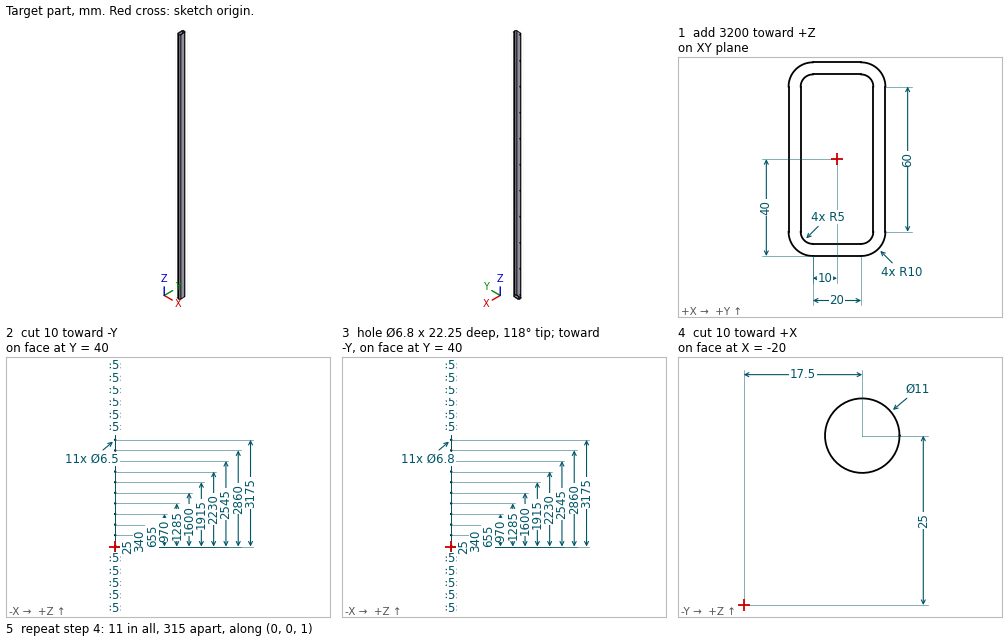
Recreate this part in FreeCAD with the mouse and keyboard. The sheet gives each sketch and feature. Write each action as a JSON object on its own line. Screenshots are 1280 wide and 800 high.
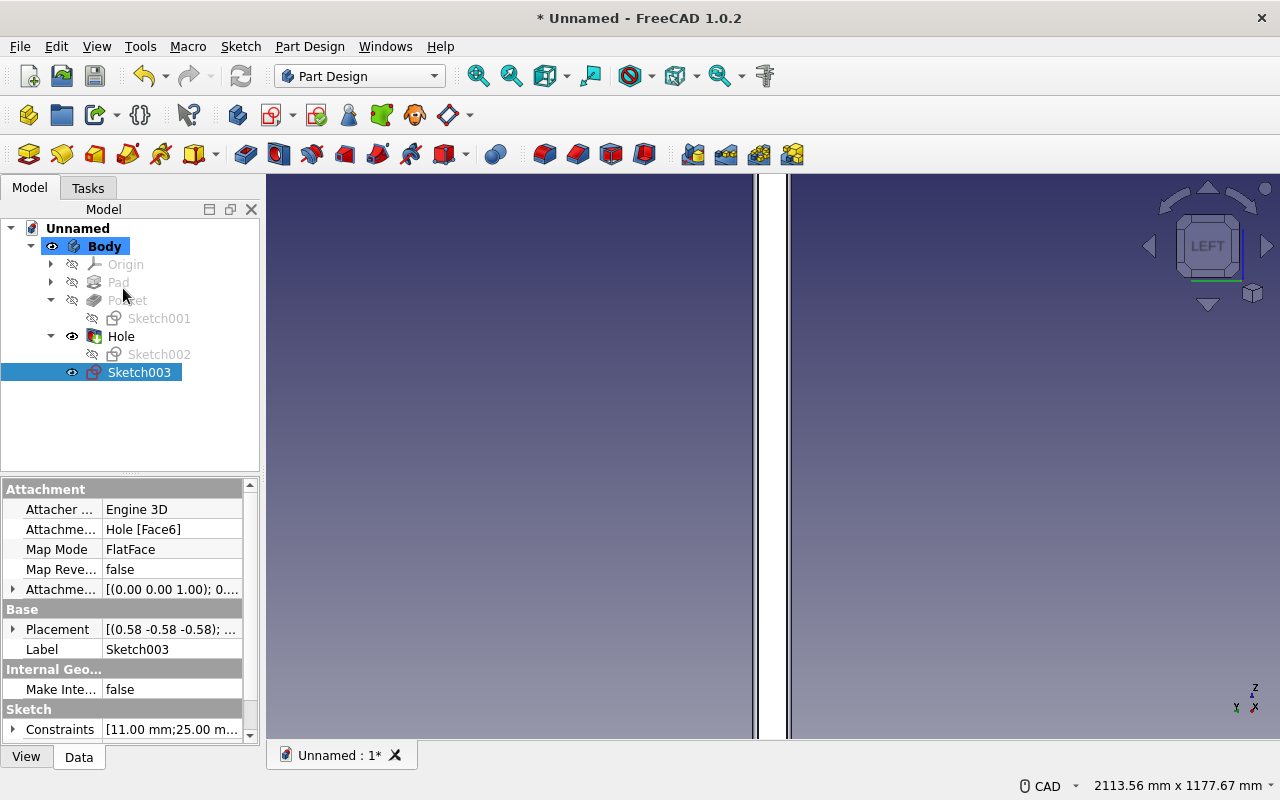
{"action": "left_click", "coordinate": [246, 154]}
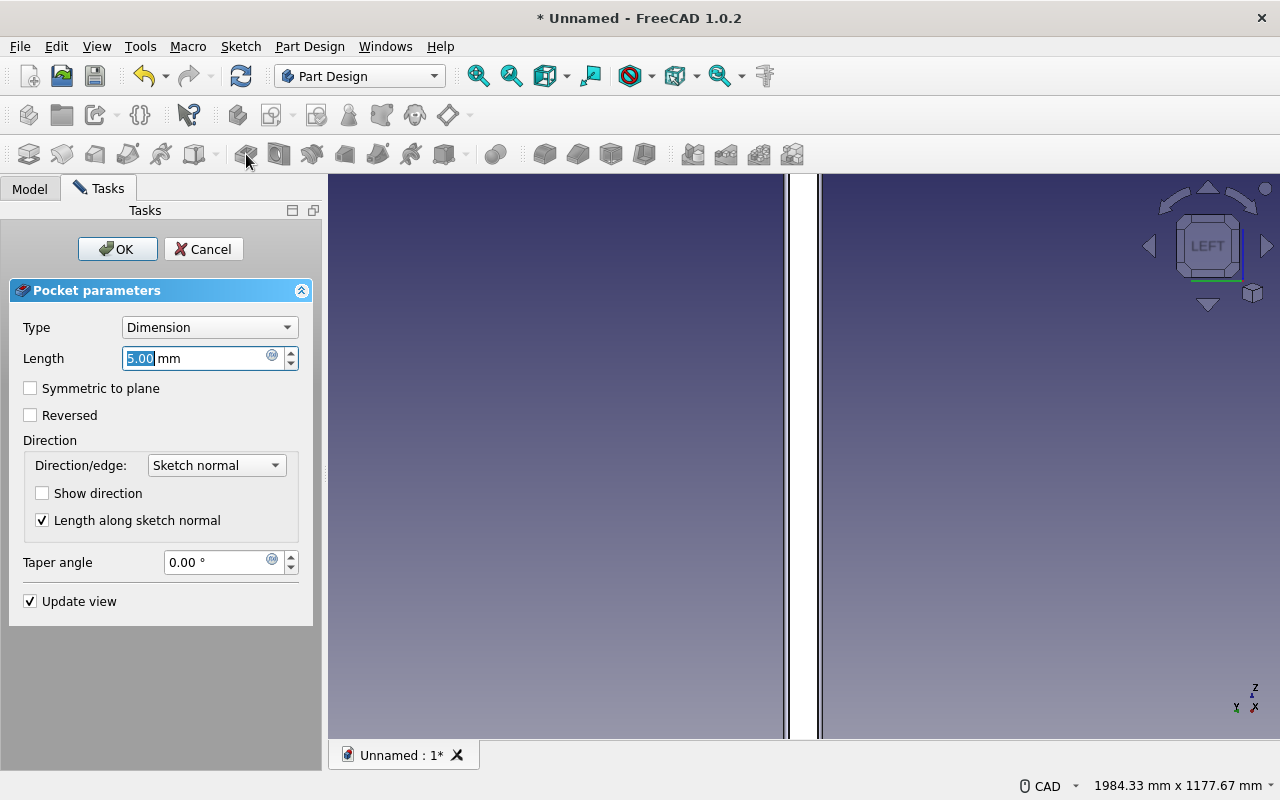
{"action": "type", "text": "10"}
{"action": "key", "text": "Tab"}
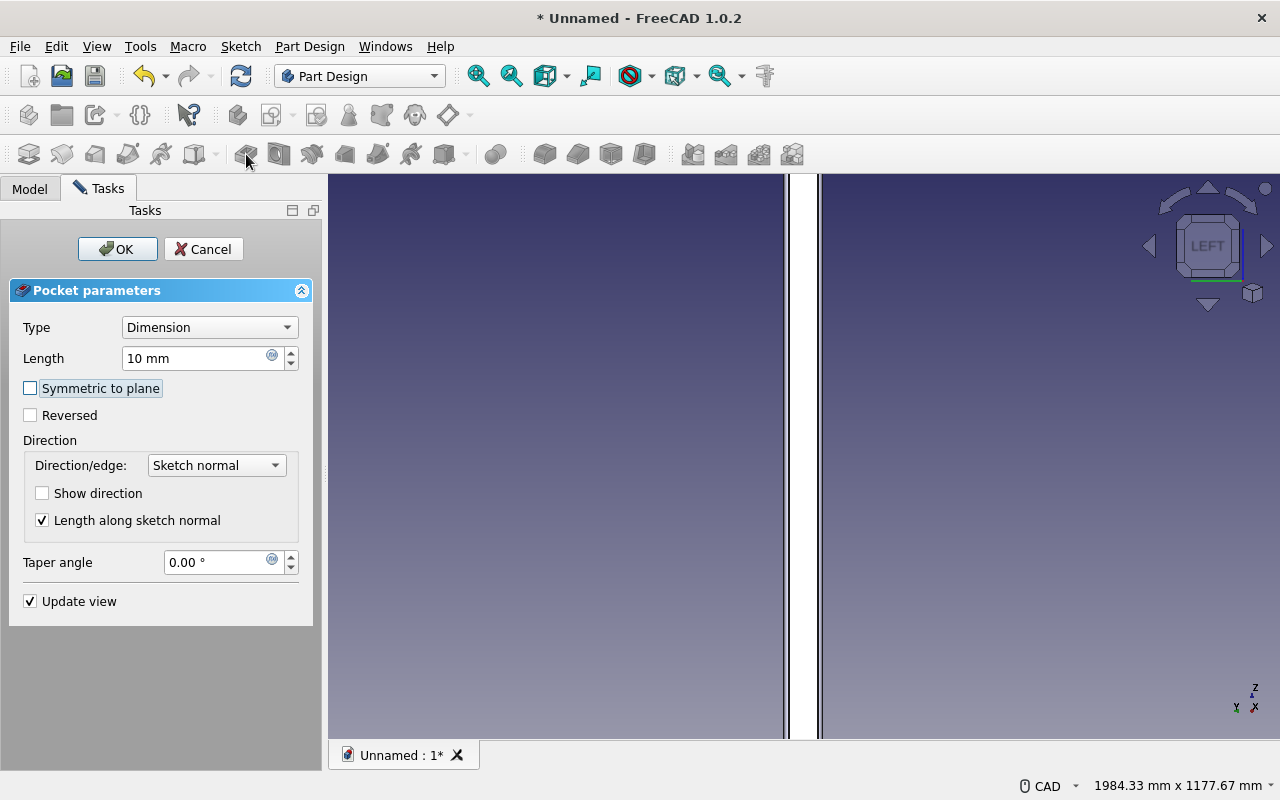
{"action": "left_click", "coordinate": [118, 249]}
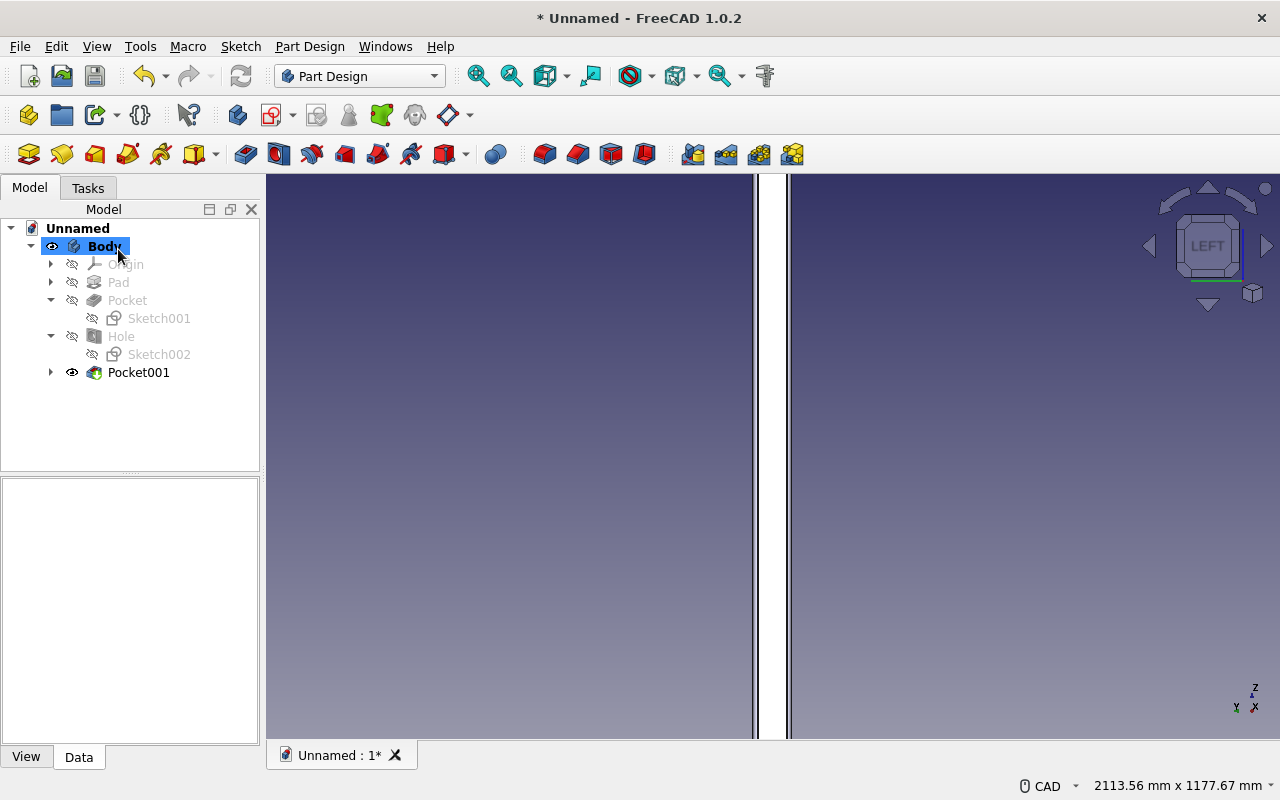
{"action": "left_click", "coordinate": [479, 76]}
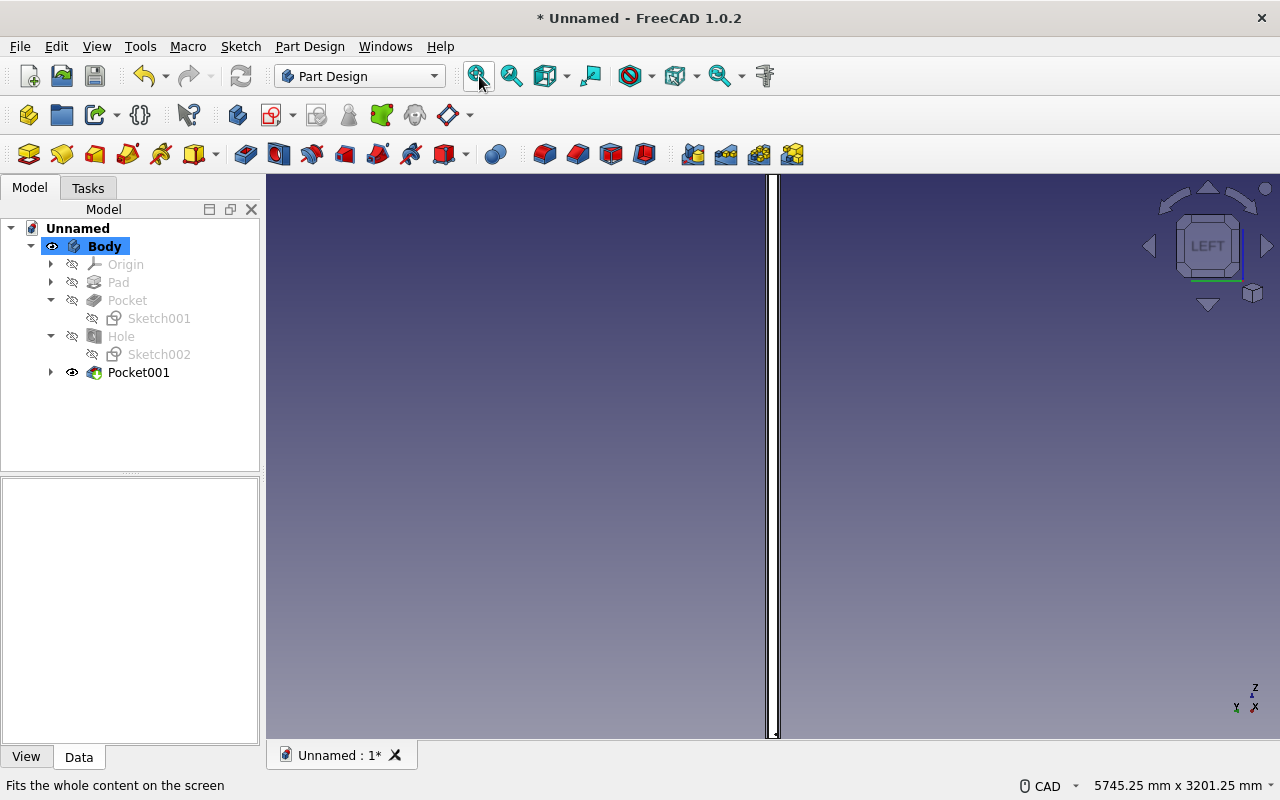
{"action": "left_click", "coordinate": [117, 372]}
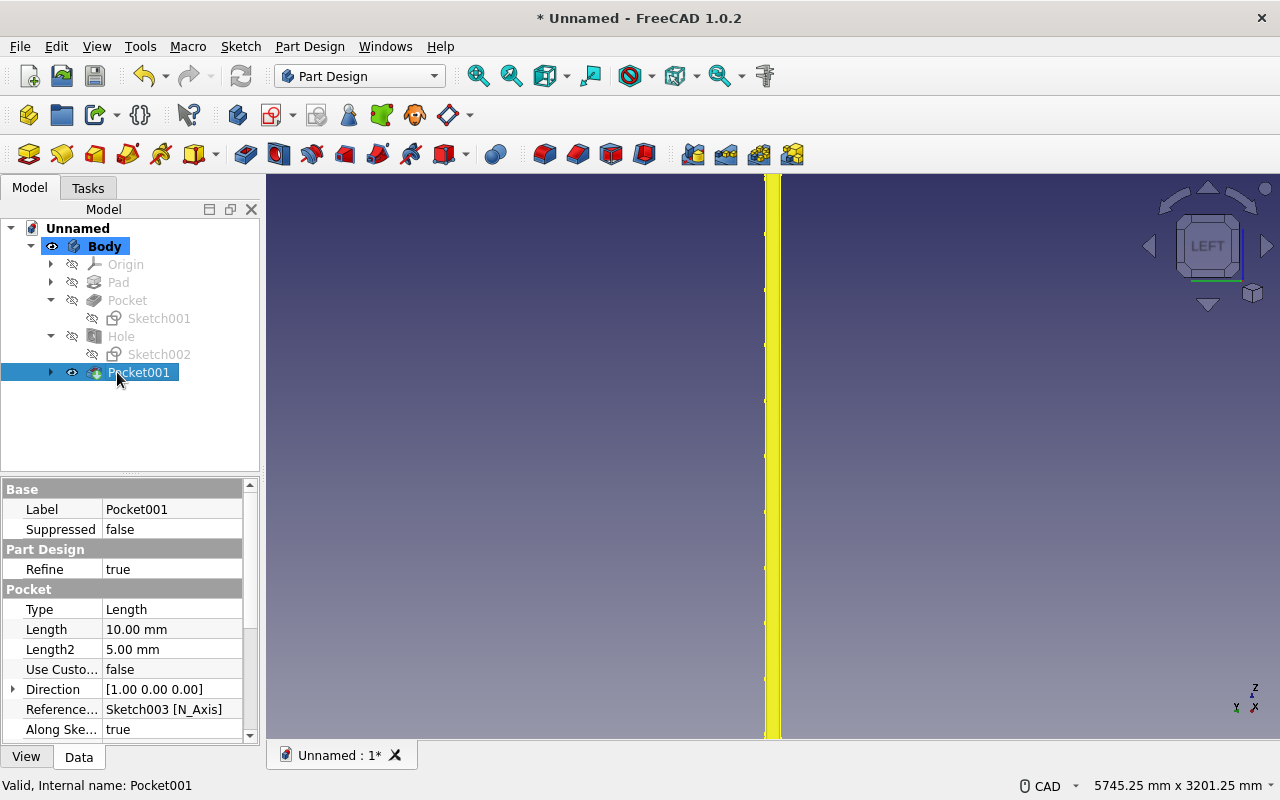
{"action": "left_click", "coordinate": [726, 154]}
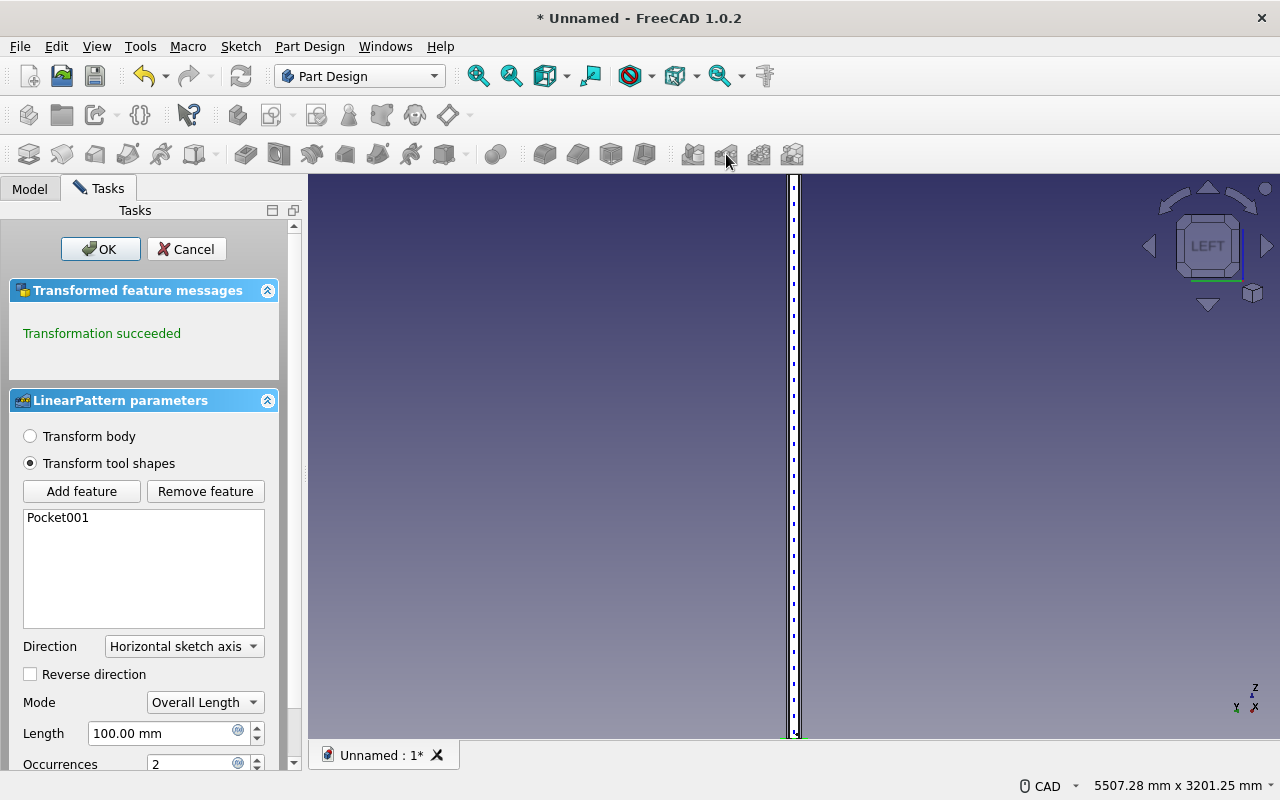
{"action": "left_click", "coordinate": [185, 646]}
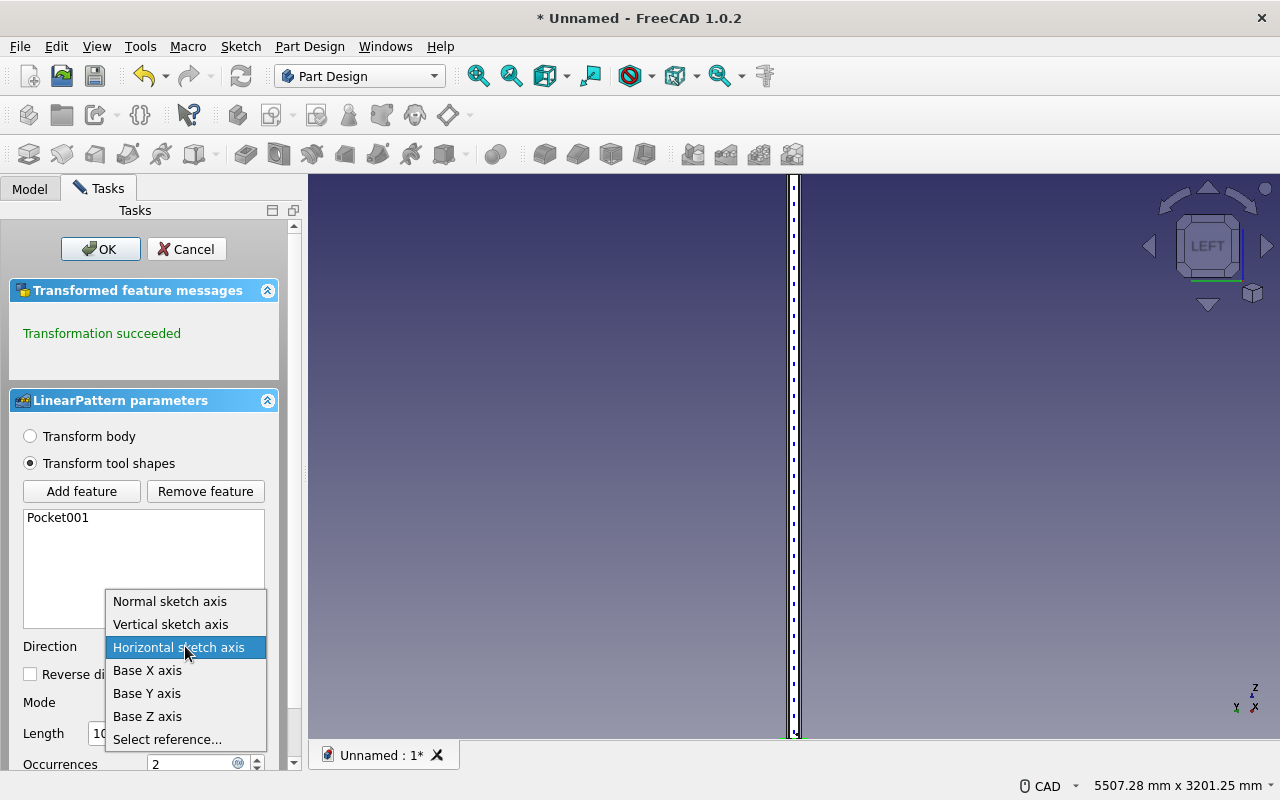
{"action": "left_click", "coordinate": [184, 716]}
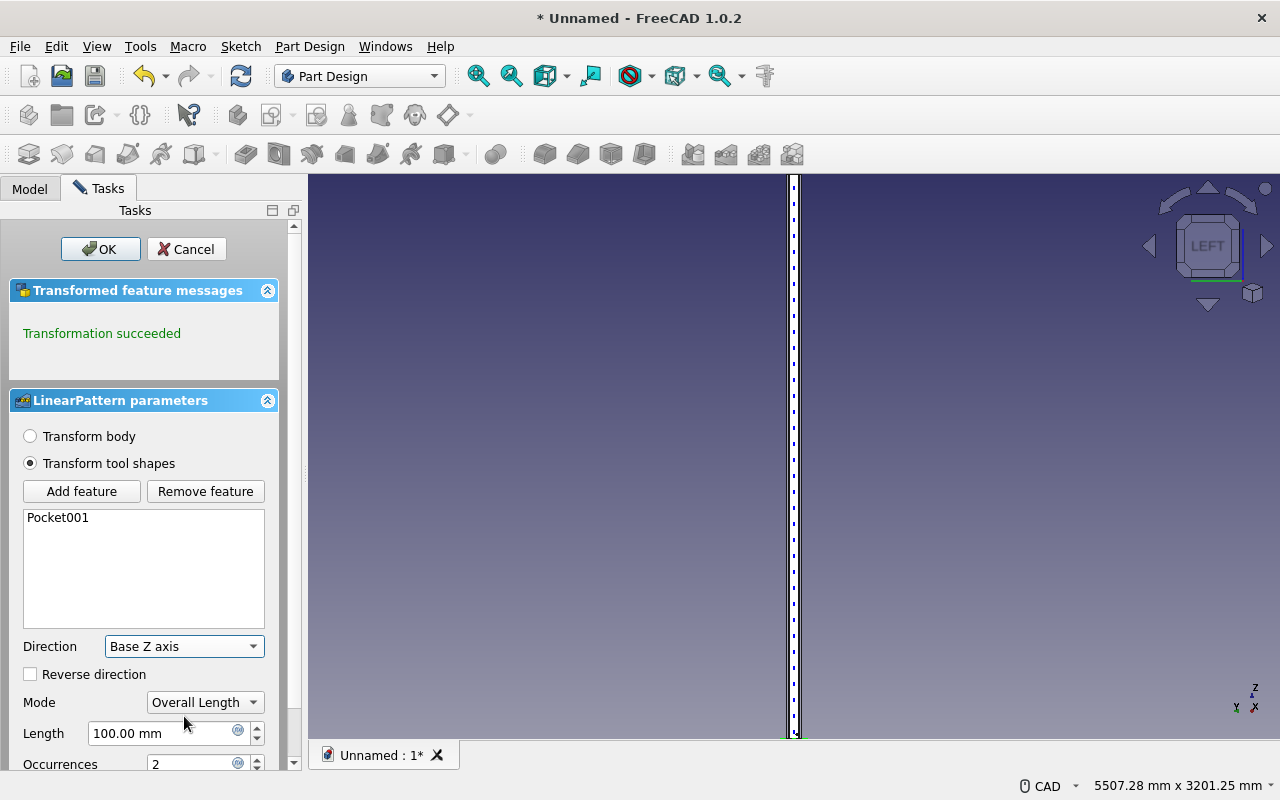
{"action": "left_click", "coordinate": [206, 702]}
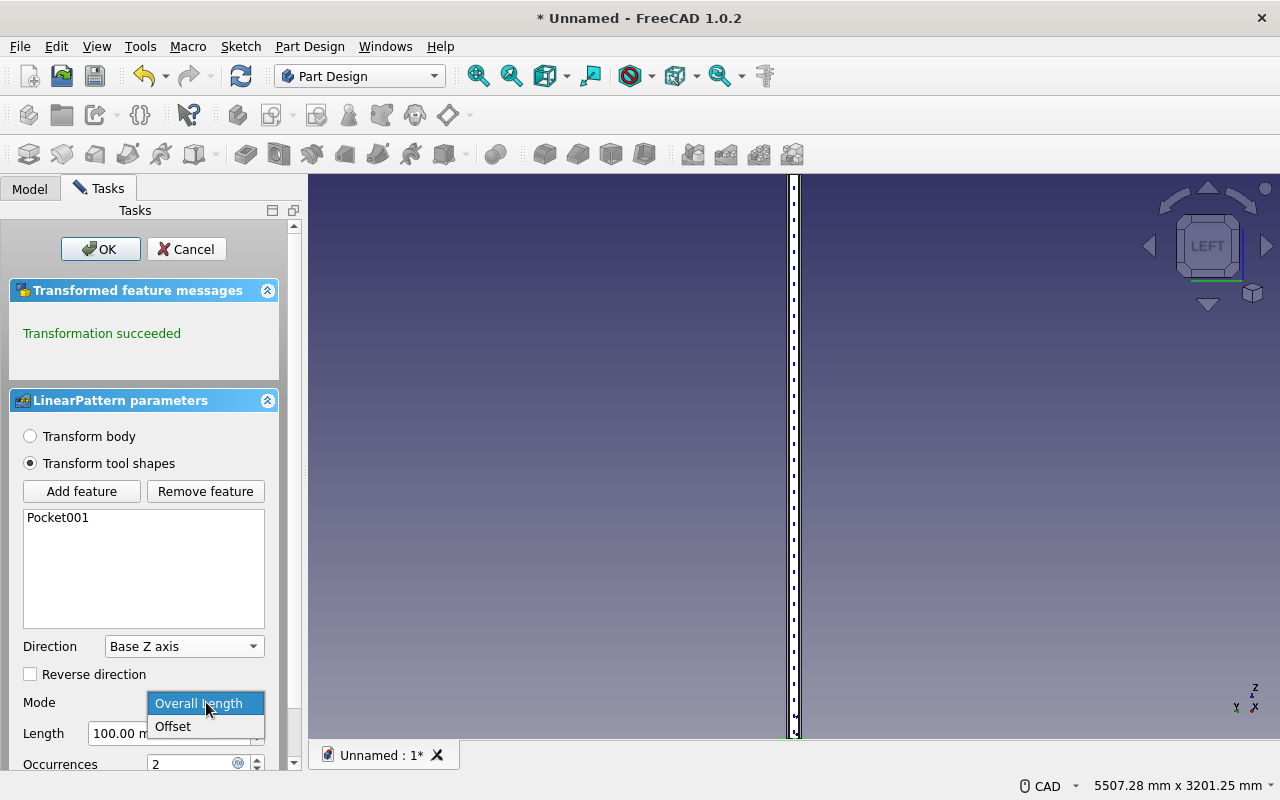
{"action": "left_click", "coordinate": [204, 726]}